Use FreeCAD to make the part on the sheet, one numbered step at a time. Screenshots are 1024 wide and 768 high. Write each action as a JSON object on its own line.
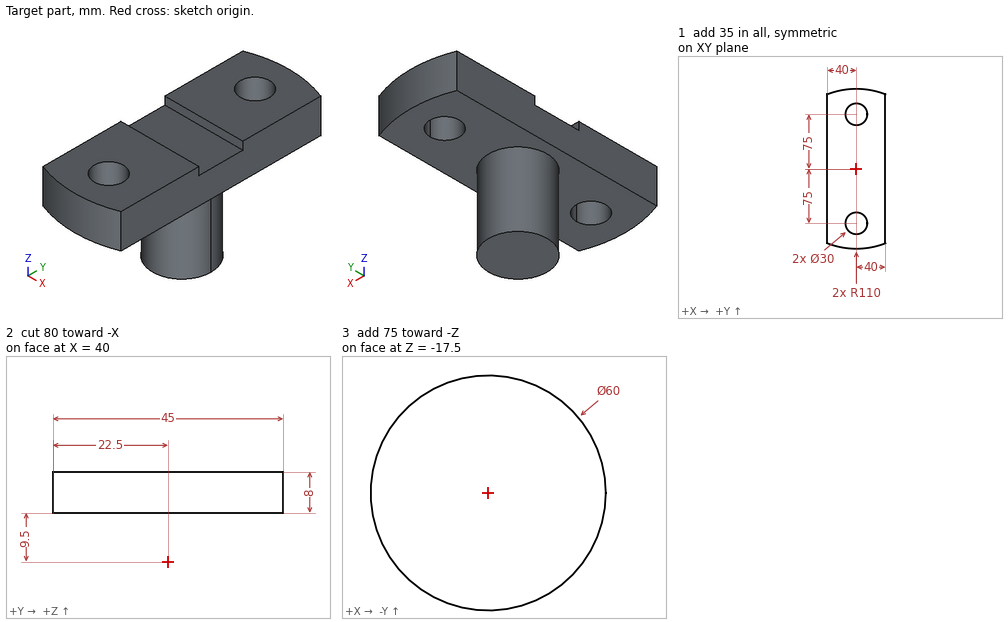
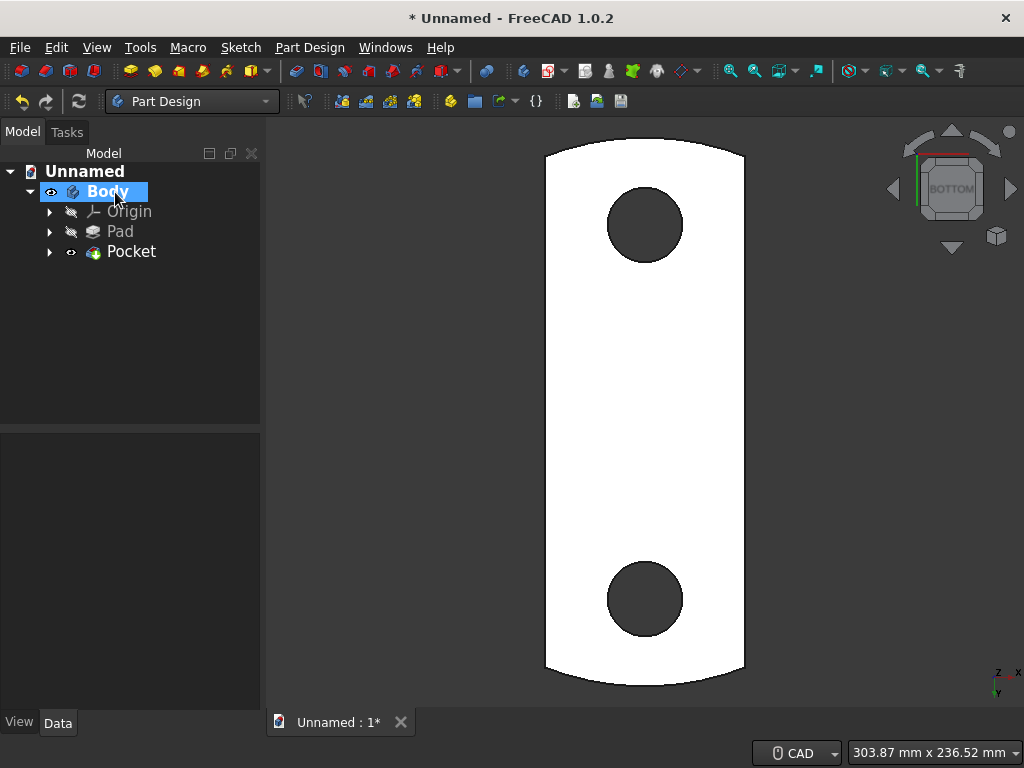
{"action": "left_click", "coordinate": [645, 411]}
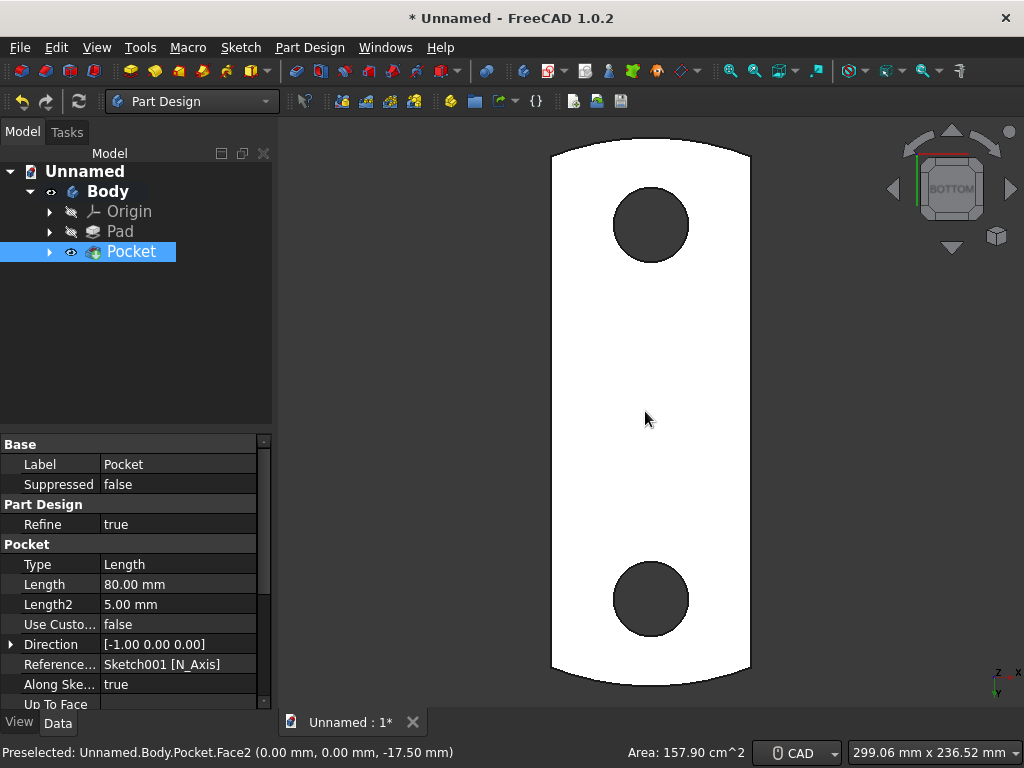
{"action": "left_click", "coordinate": [548, 72]}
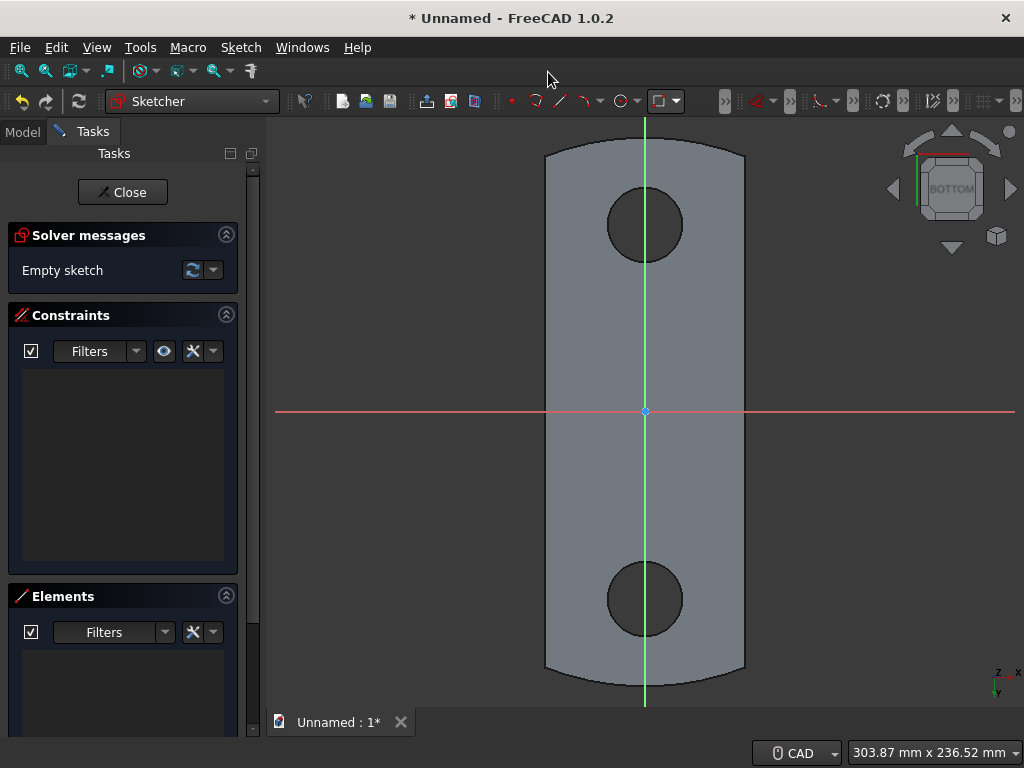
{"action": "scroll", "coordinate": [685, 412], "scroll_direction": "up", "scroll_amount": 5}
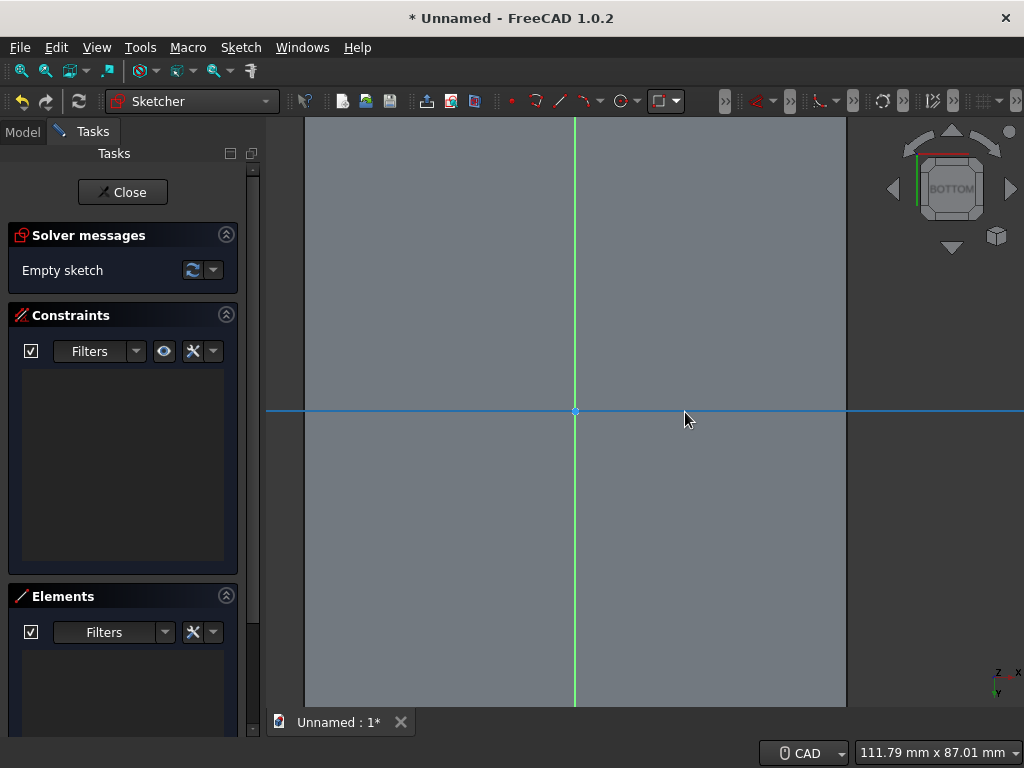
{"action": "left_click", "coordinate": [622, 102]}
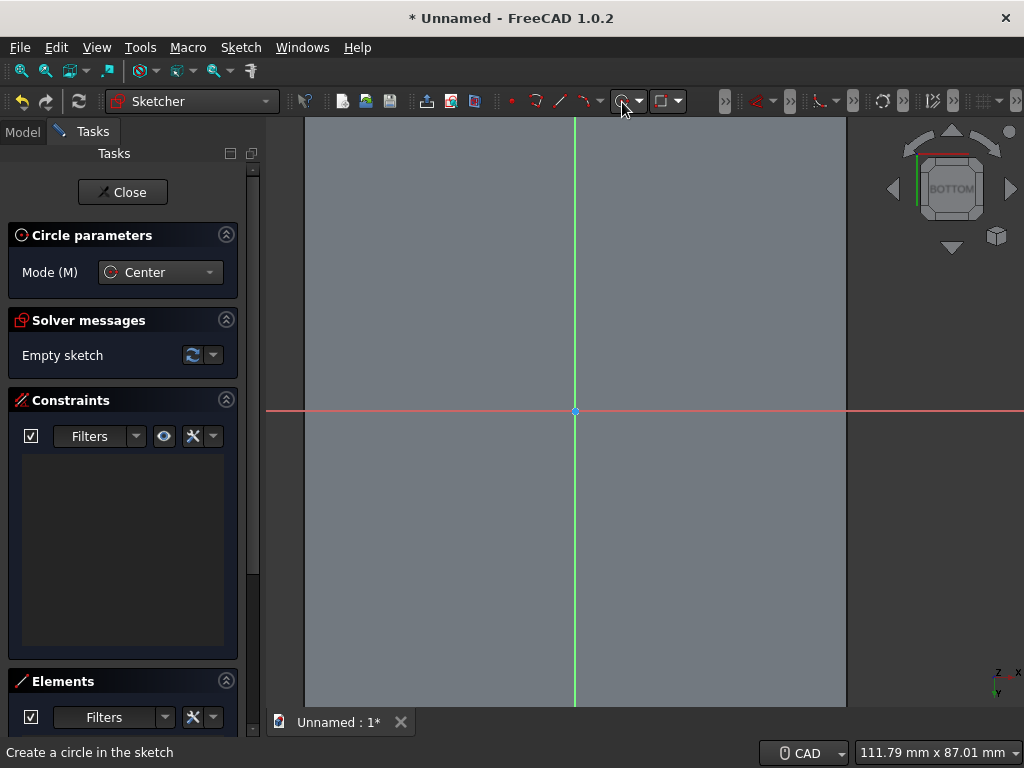
{"action": "left_click", "coordinate": [575, 411]}
{"action": "mouse_move", "coordinate": [719, 267]}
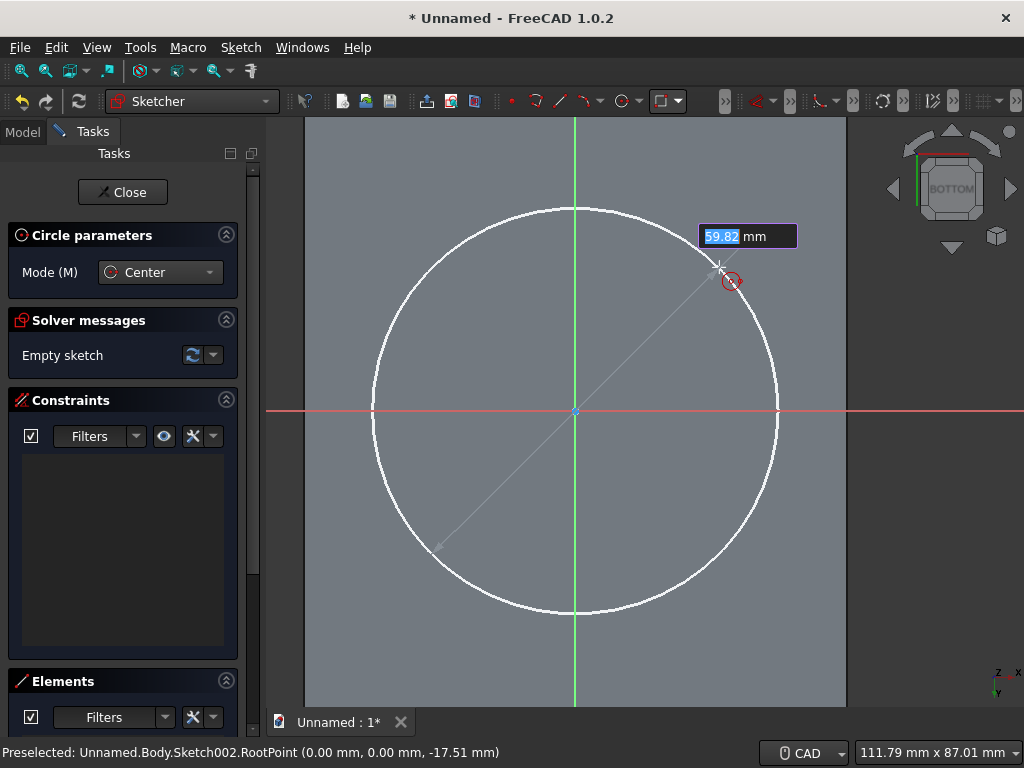
{"action": "type", "text": "60"}
{"action": "key", "text": "Return"}
{"action": "key", "text": "Escape"}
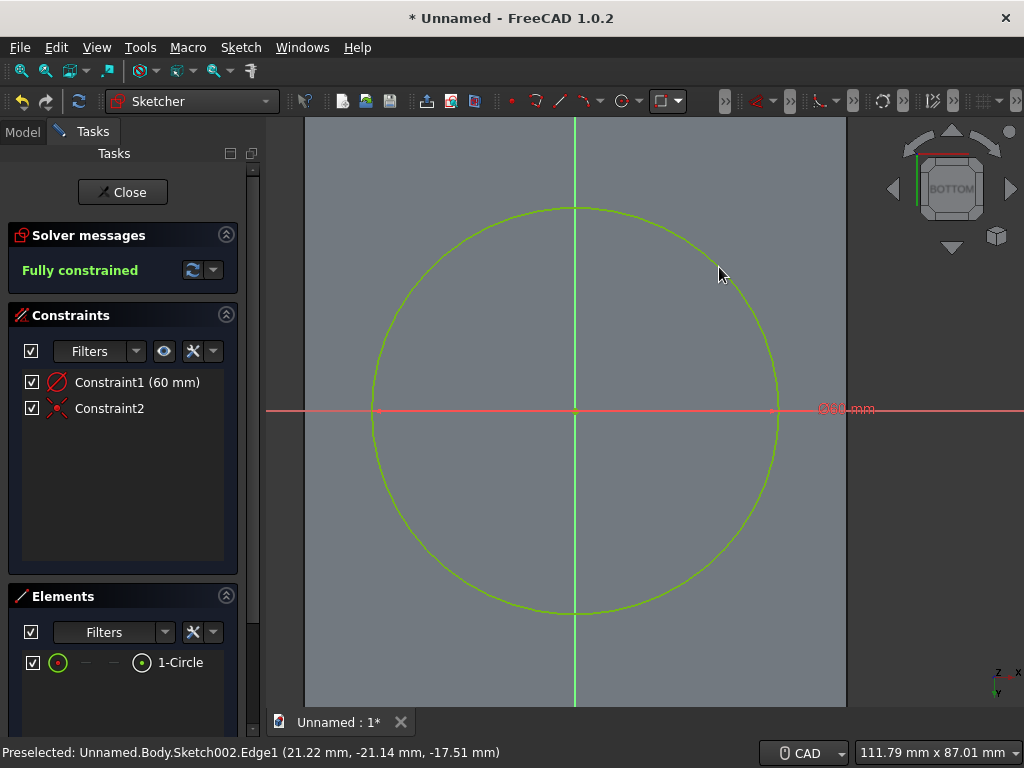
{"action": "left_click", "coordinate": [123, 192]}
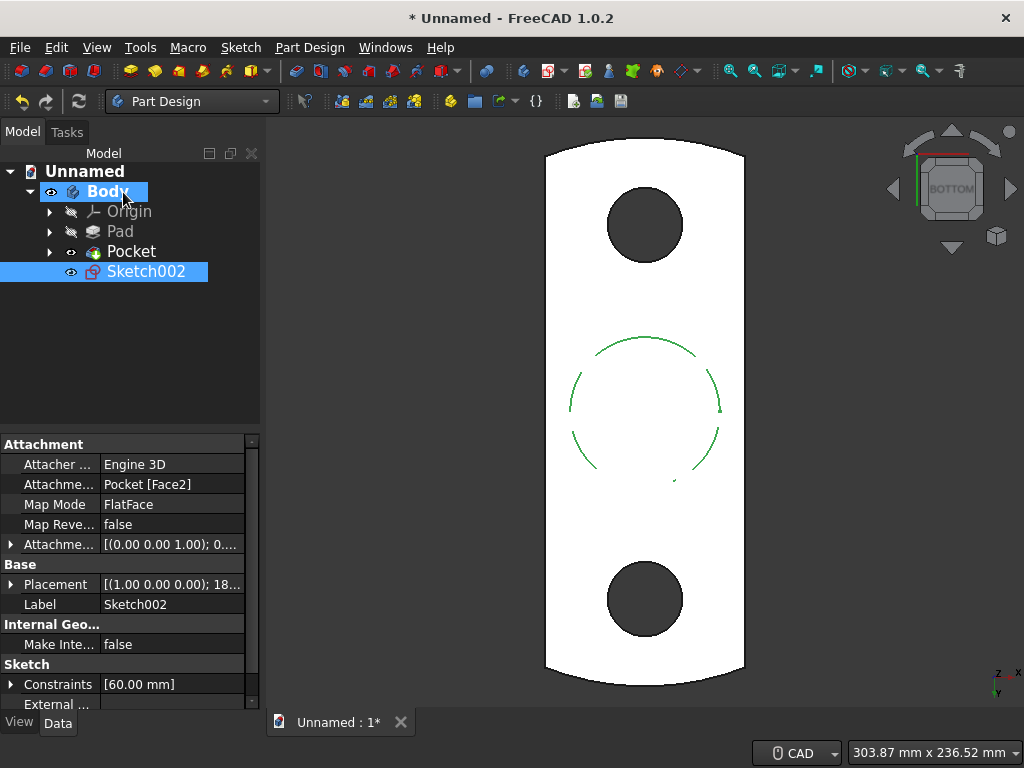
{"action": "left_click", "coordinate": [132, 72]}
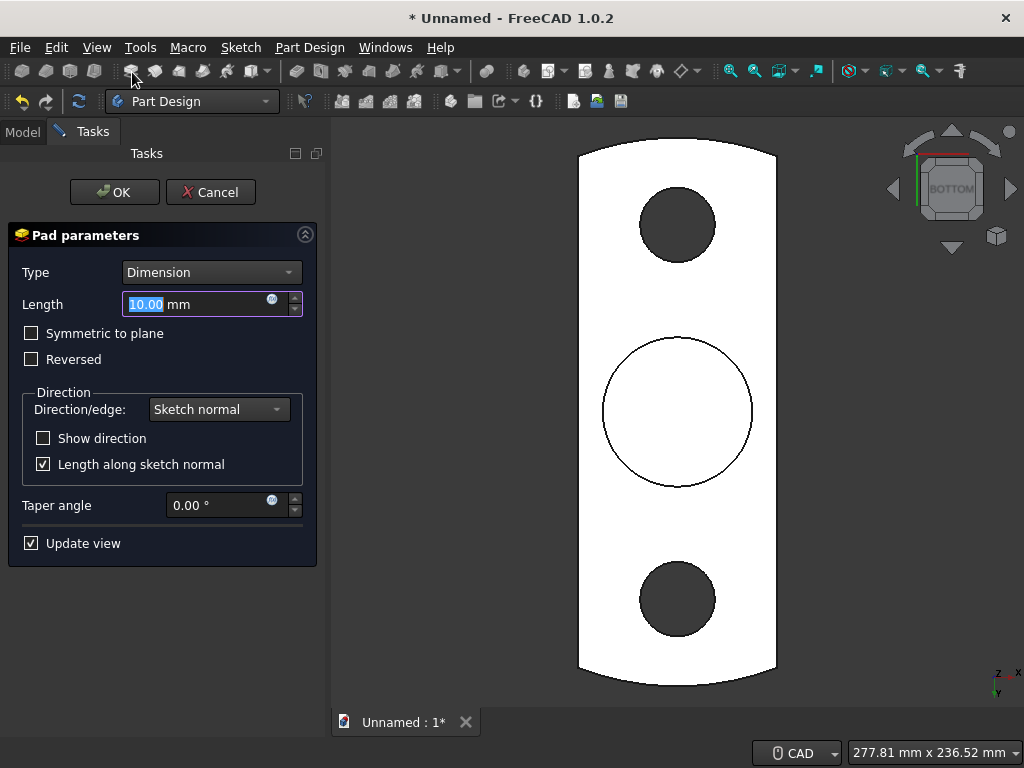
{"action": "type", "text": "75"}
{"action": "key", "text": "Tab"}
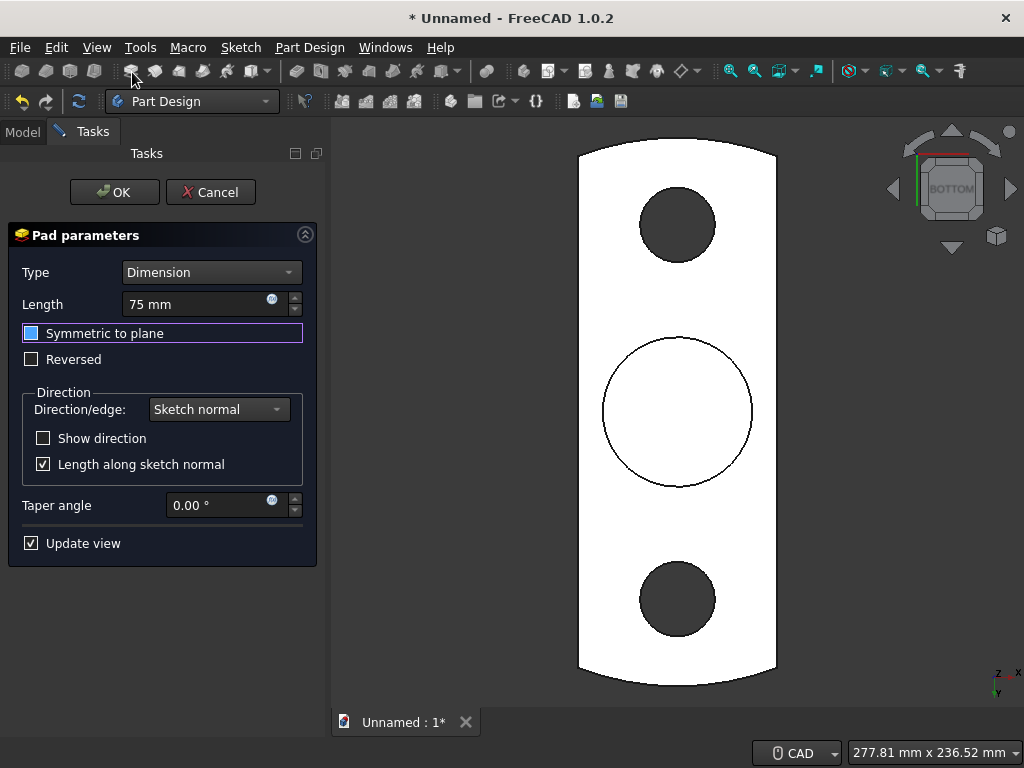
{"action": "left_click", "coordinate": [115, 192]}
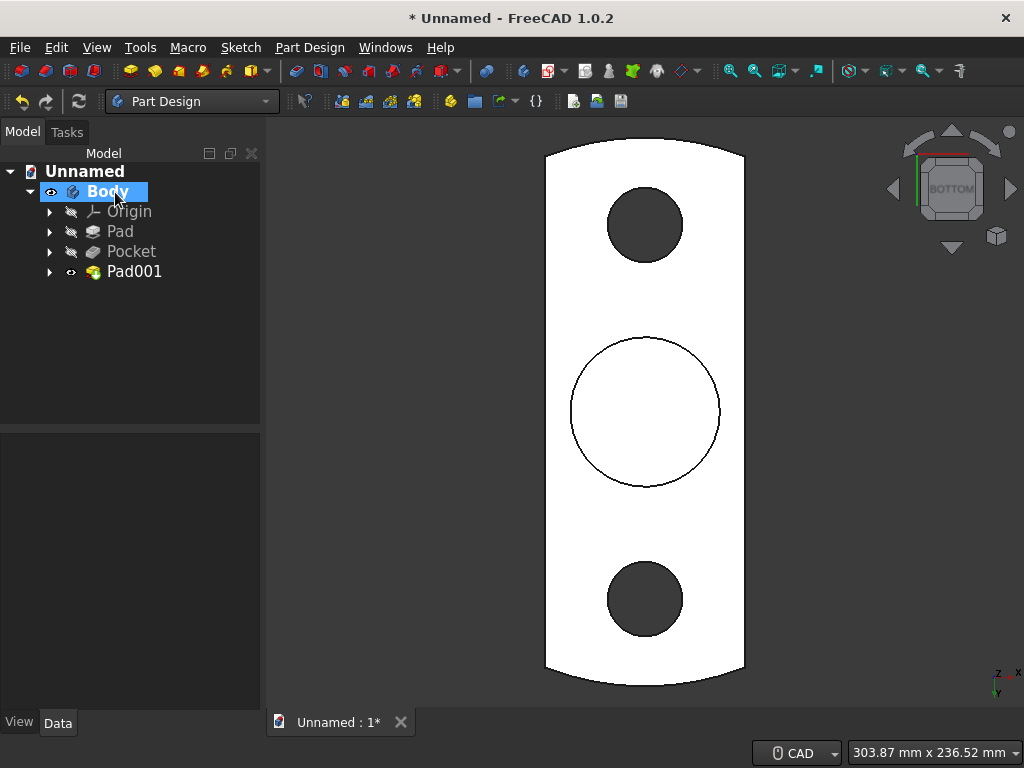
{"action": "key", "text": "0"}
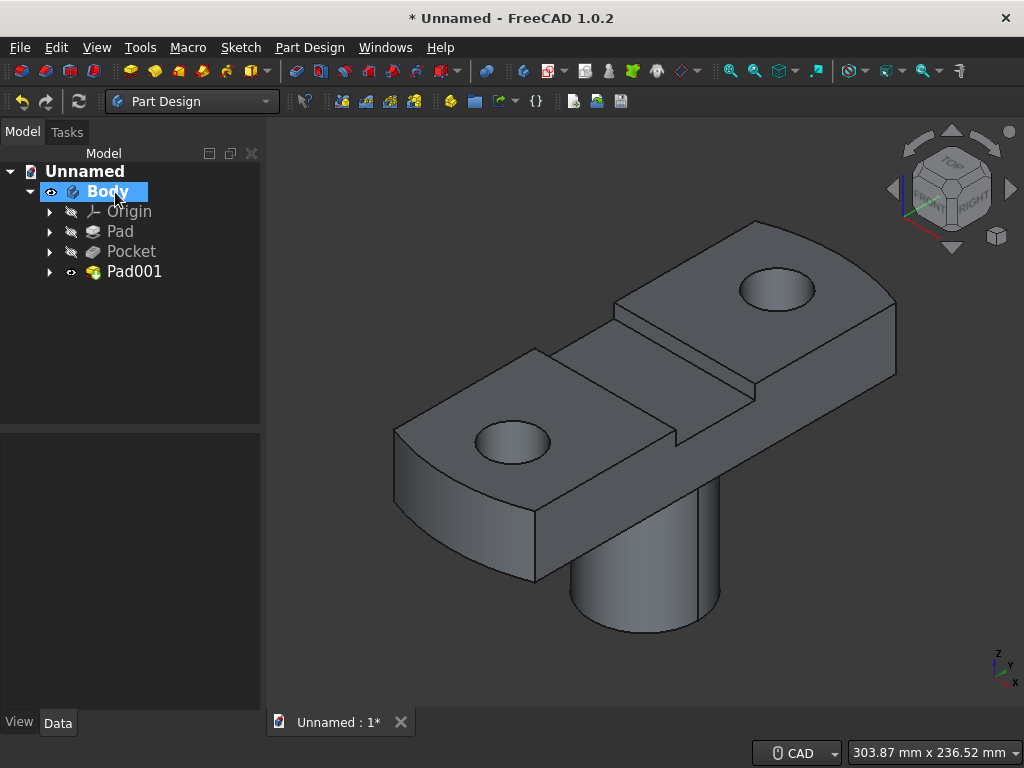
{"action": "key", "text": "v f"}